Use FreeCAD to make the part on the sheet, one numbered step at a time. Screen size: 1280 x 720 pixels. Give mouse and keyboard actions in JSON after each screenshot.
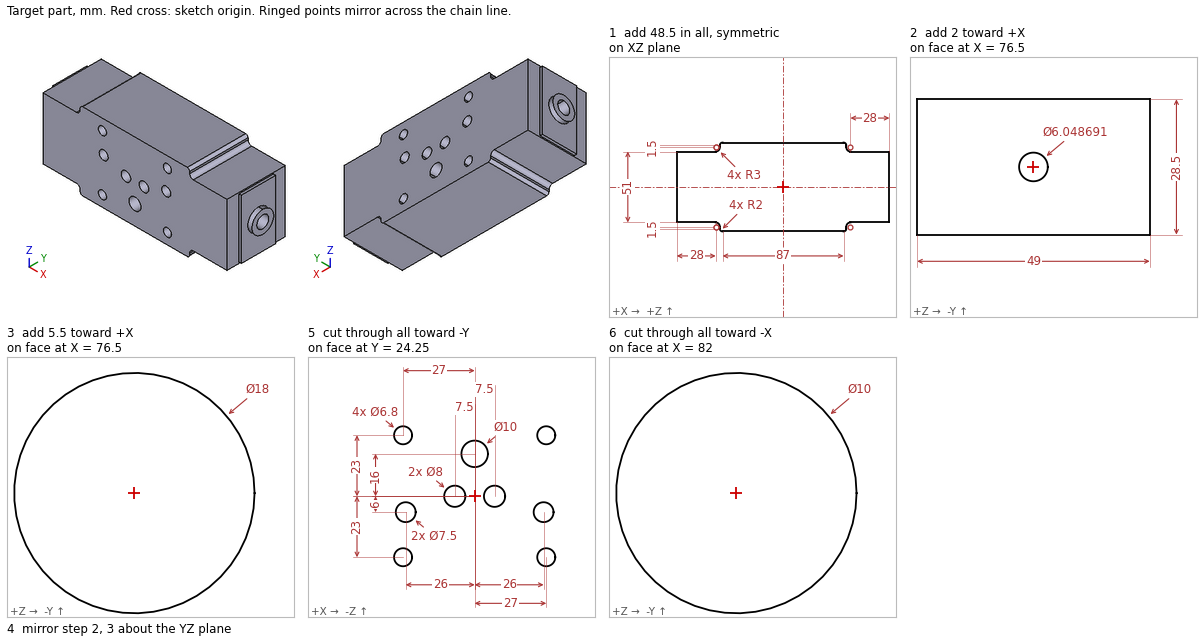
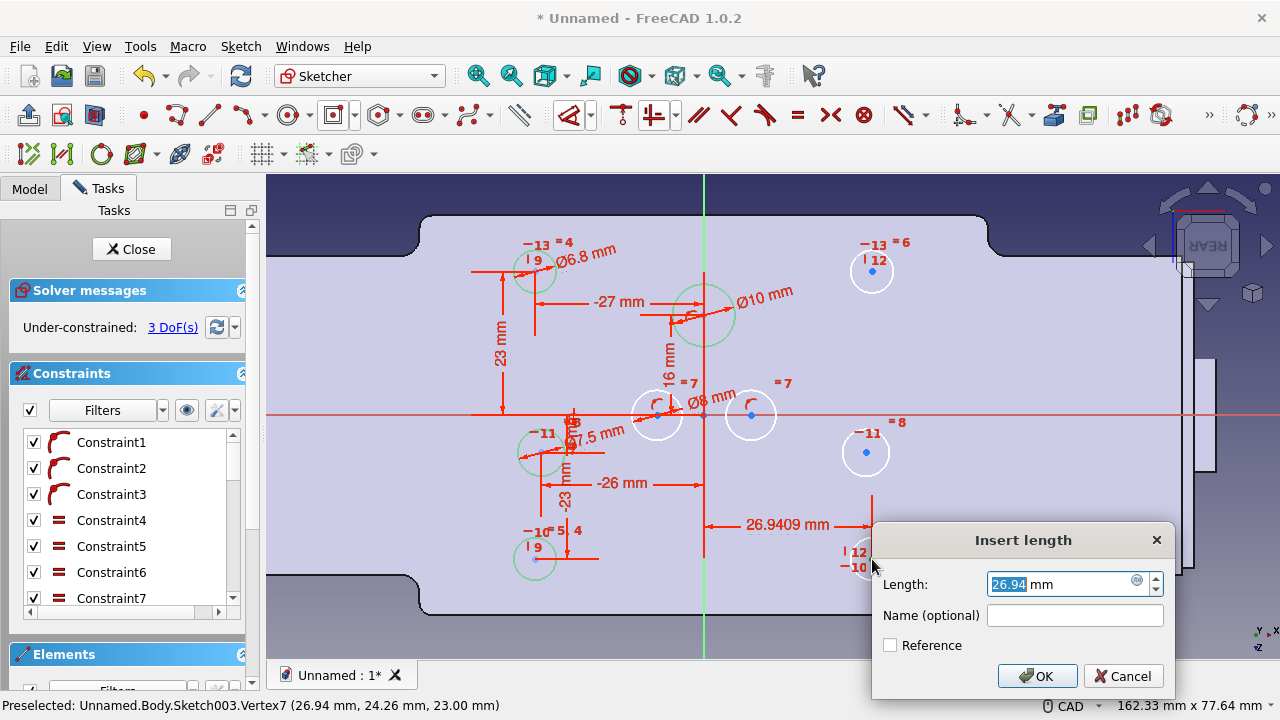
{"action": "type", "text": "27"}
{"action": "key", "text": "Return"}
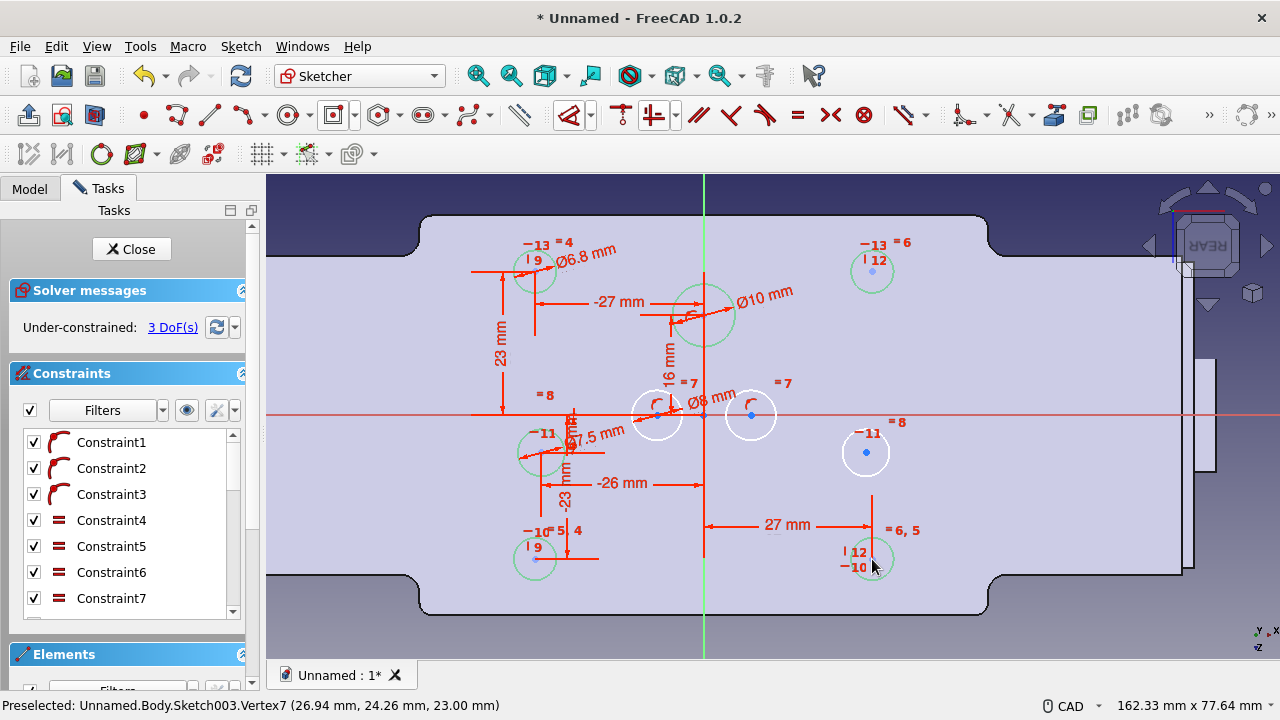
{"action": "left_click", "coordinate": [866, 453]}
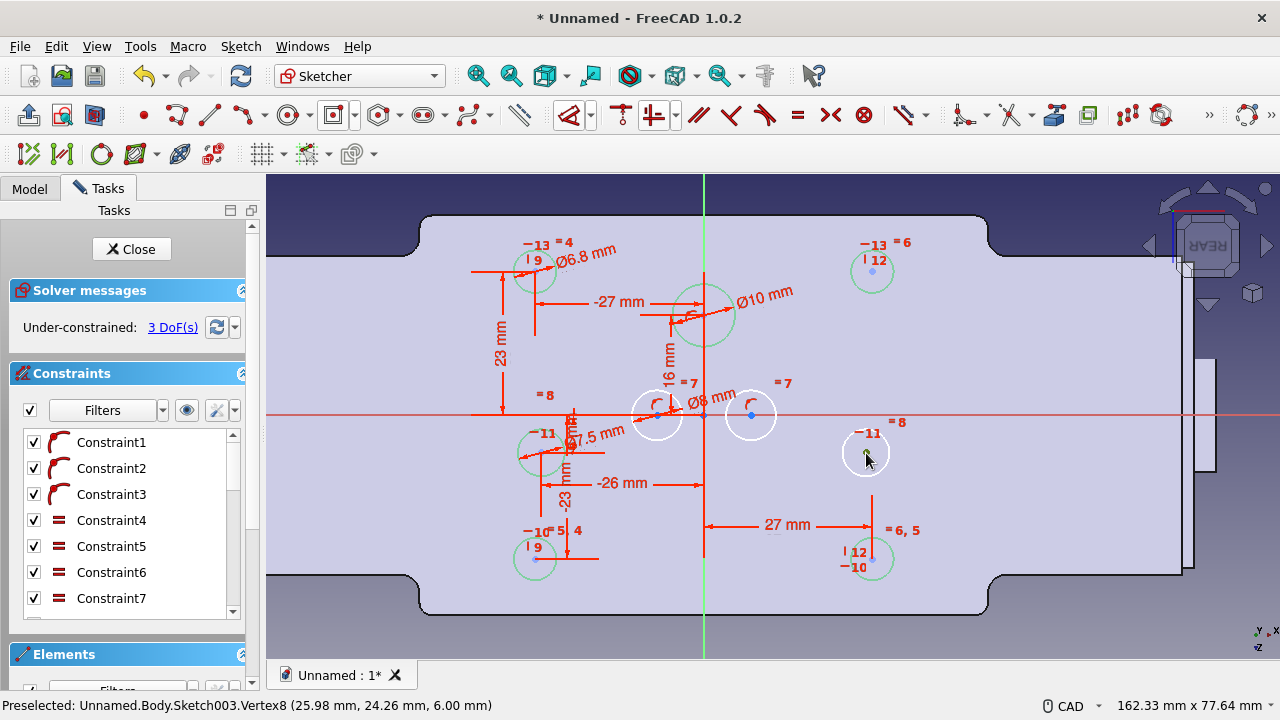
{"action": "key", "text": "l"}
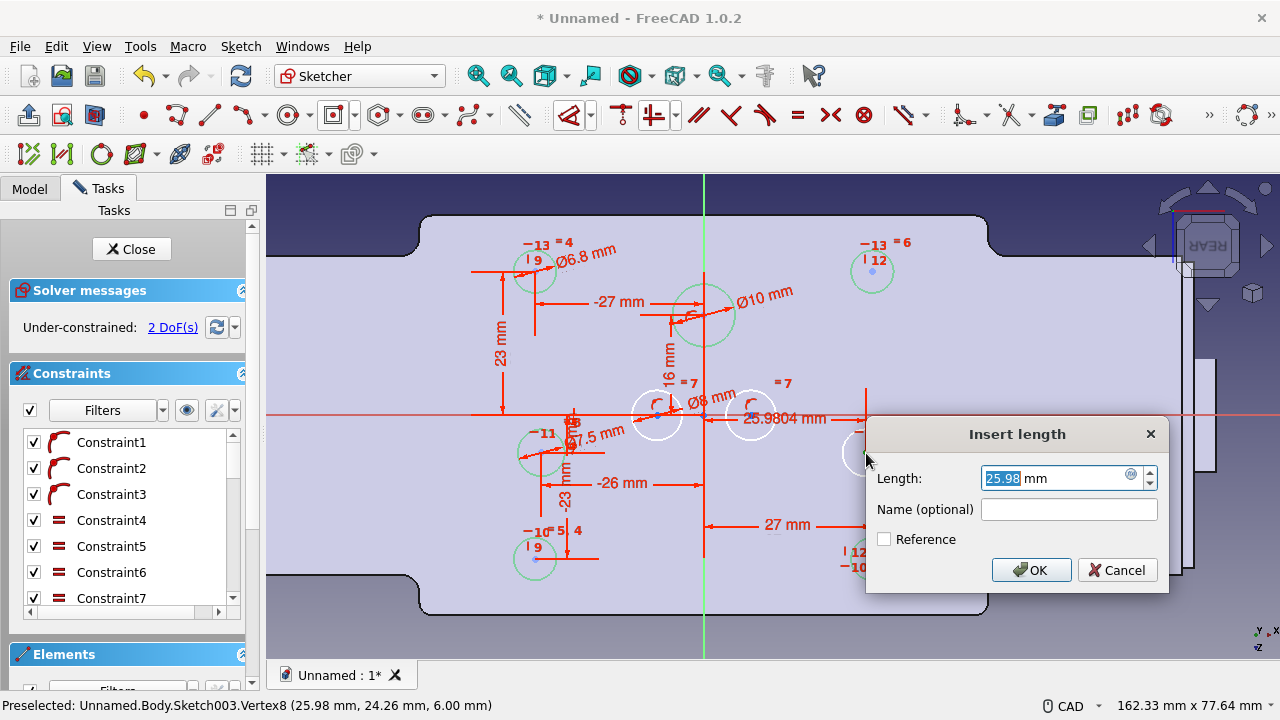
{"action": "type", "text": "26"}
{"action": "key", "text": "Return"}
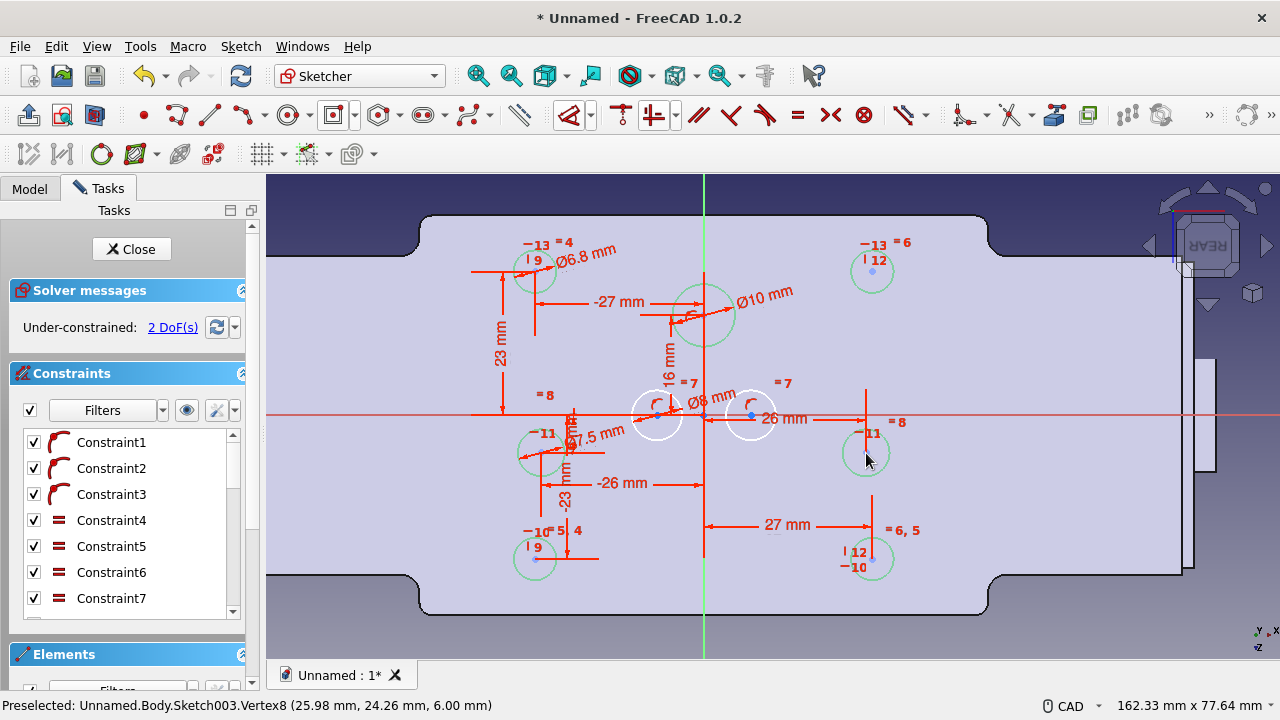
{"action": "left_click", "coordinate": [657, 415]}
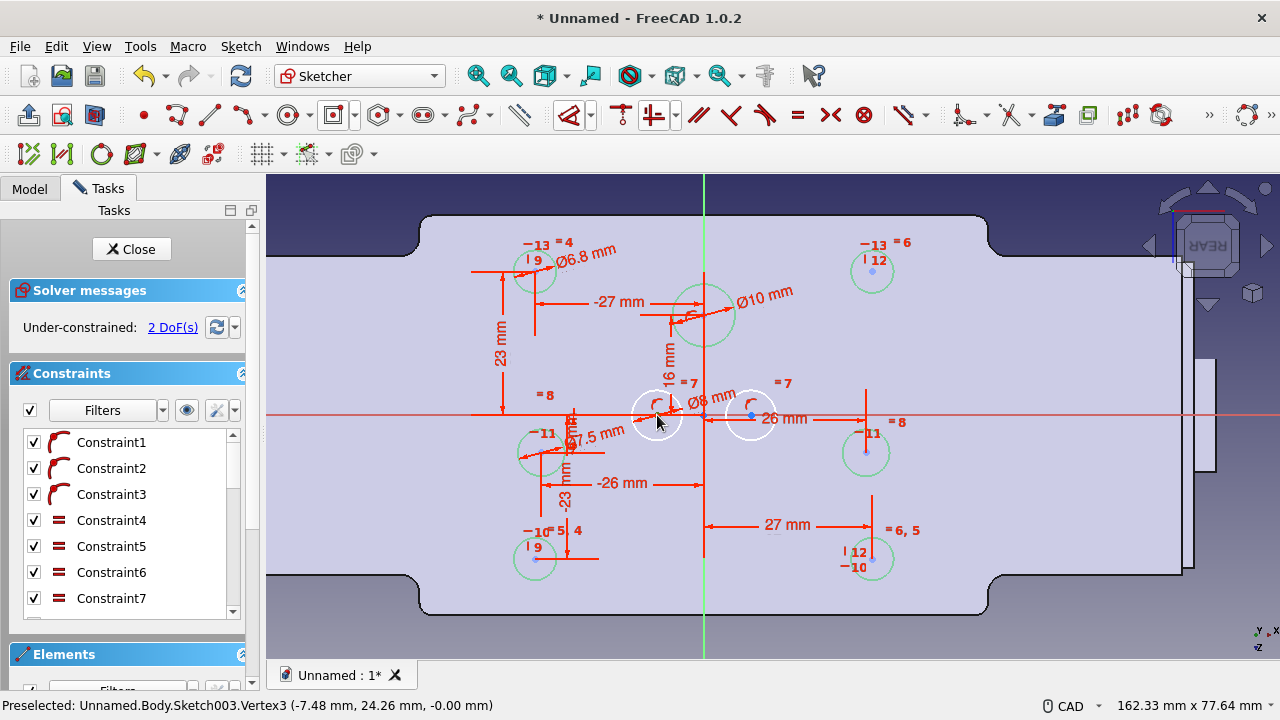
{"action": "key", "text": "l"}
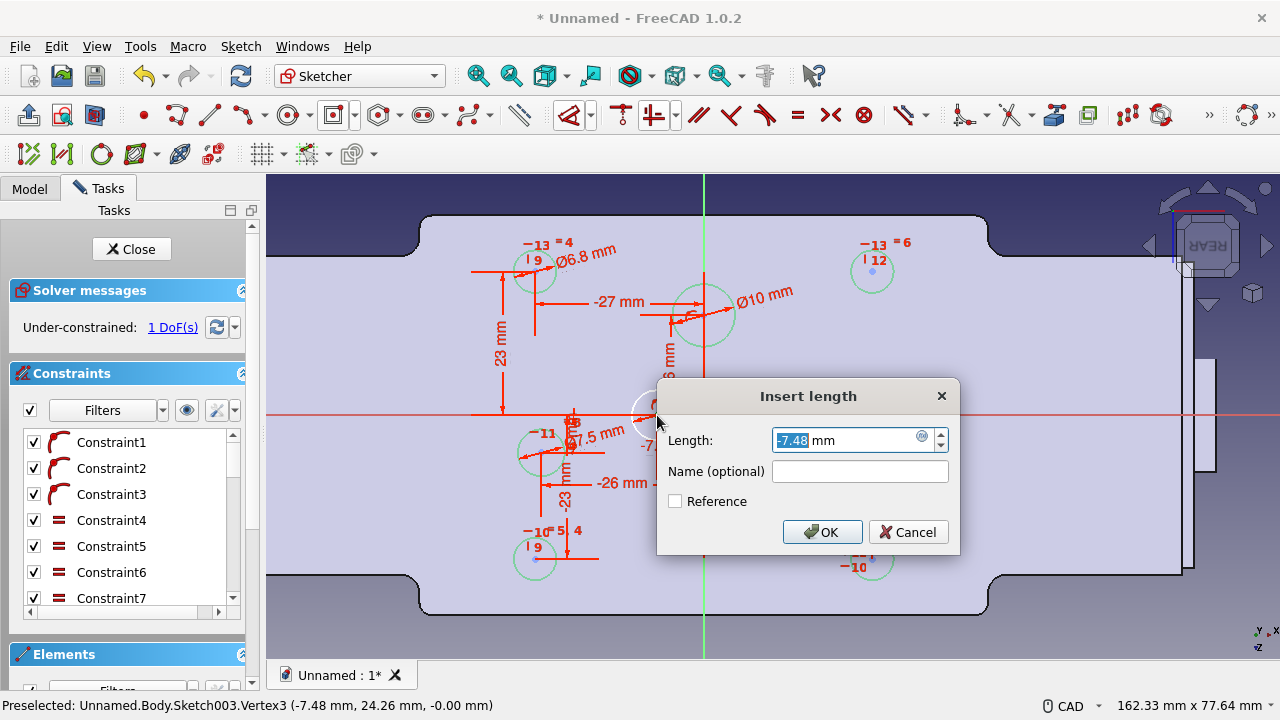
{"action": "type", "text": "-7.5"}
{"action": "key", "text": "Return"}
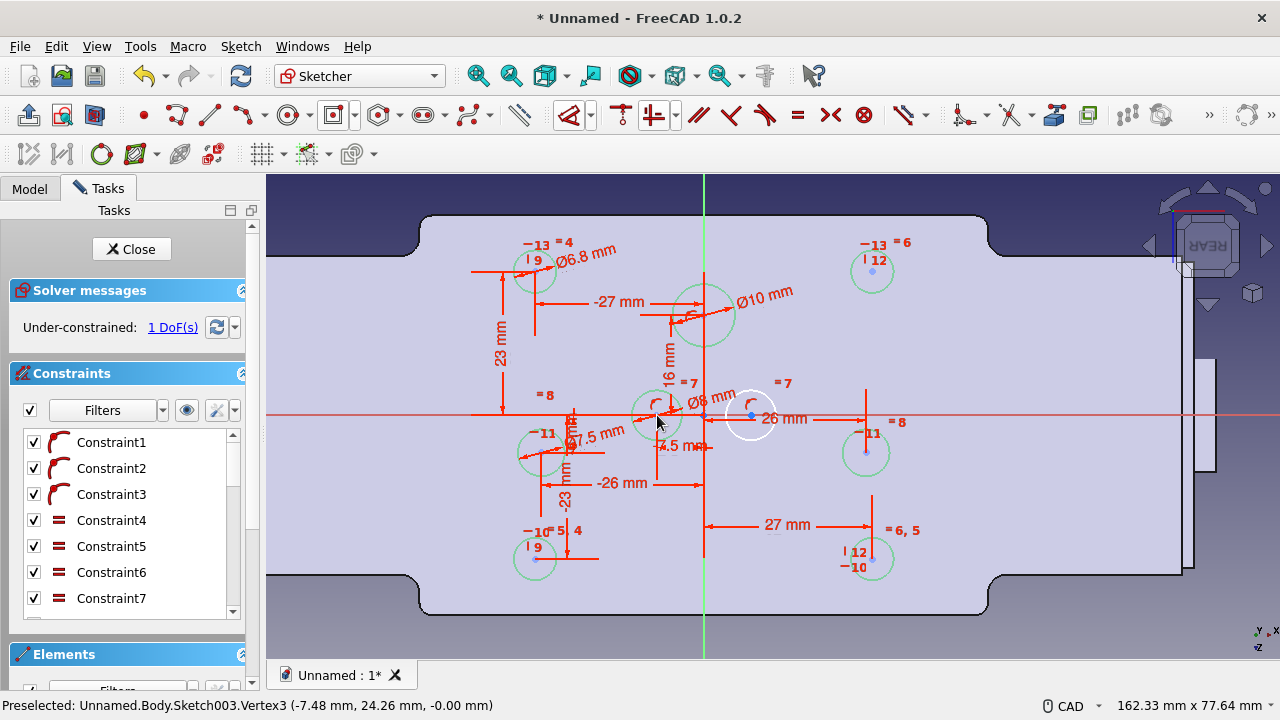
{"action": "left_click", "coordinate": [751, 415]}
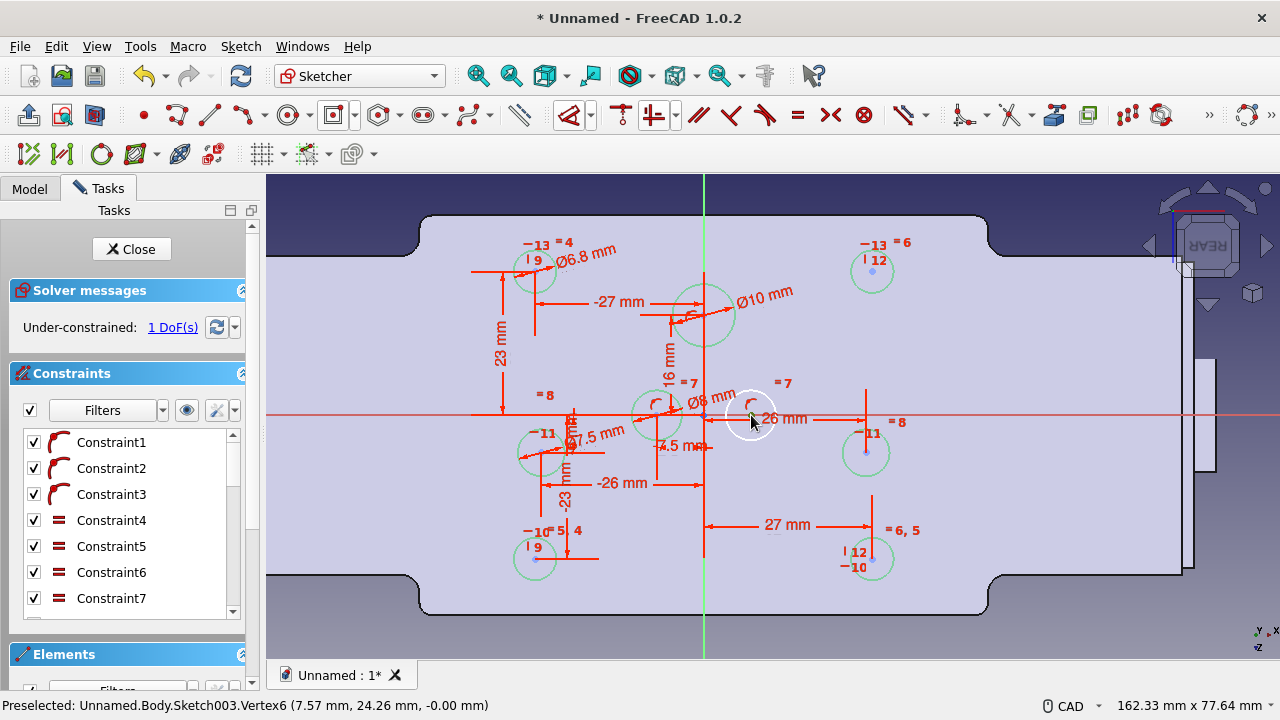
{"action": "key", "text": "l"}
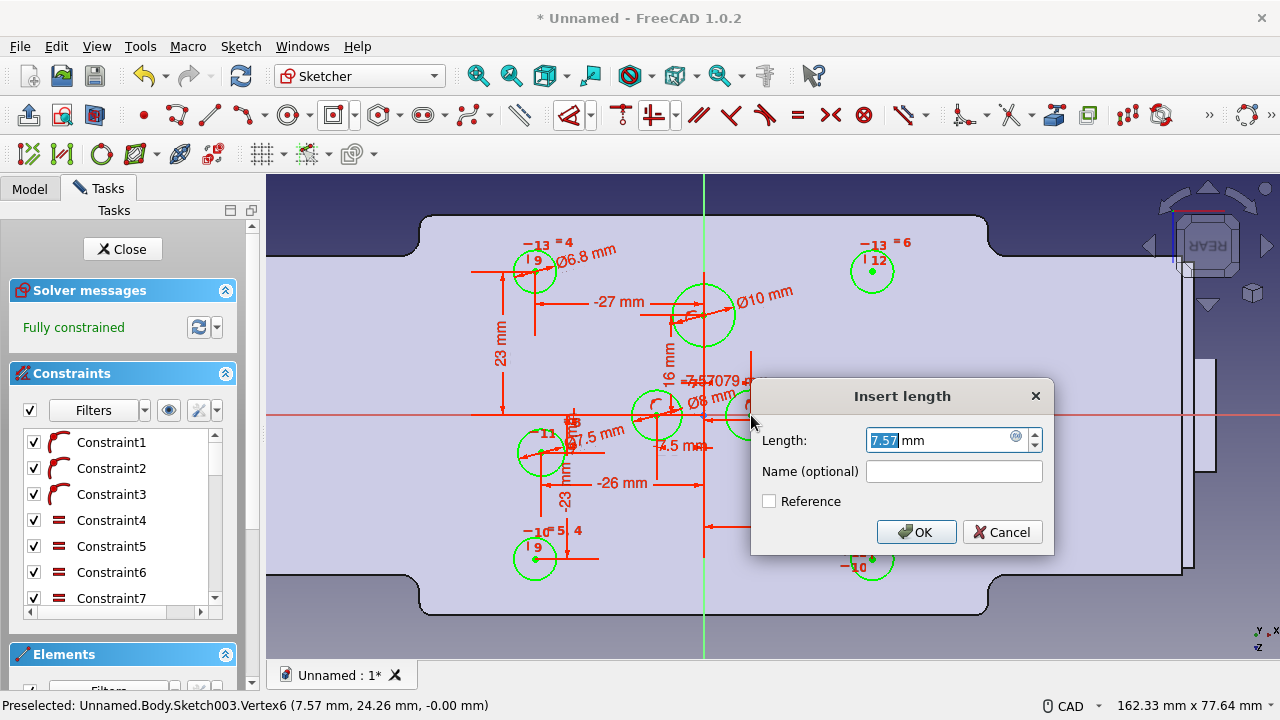
{"action": "type", "text": "7.5"}
{"action": "key", "text": "Return"}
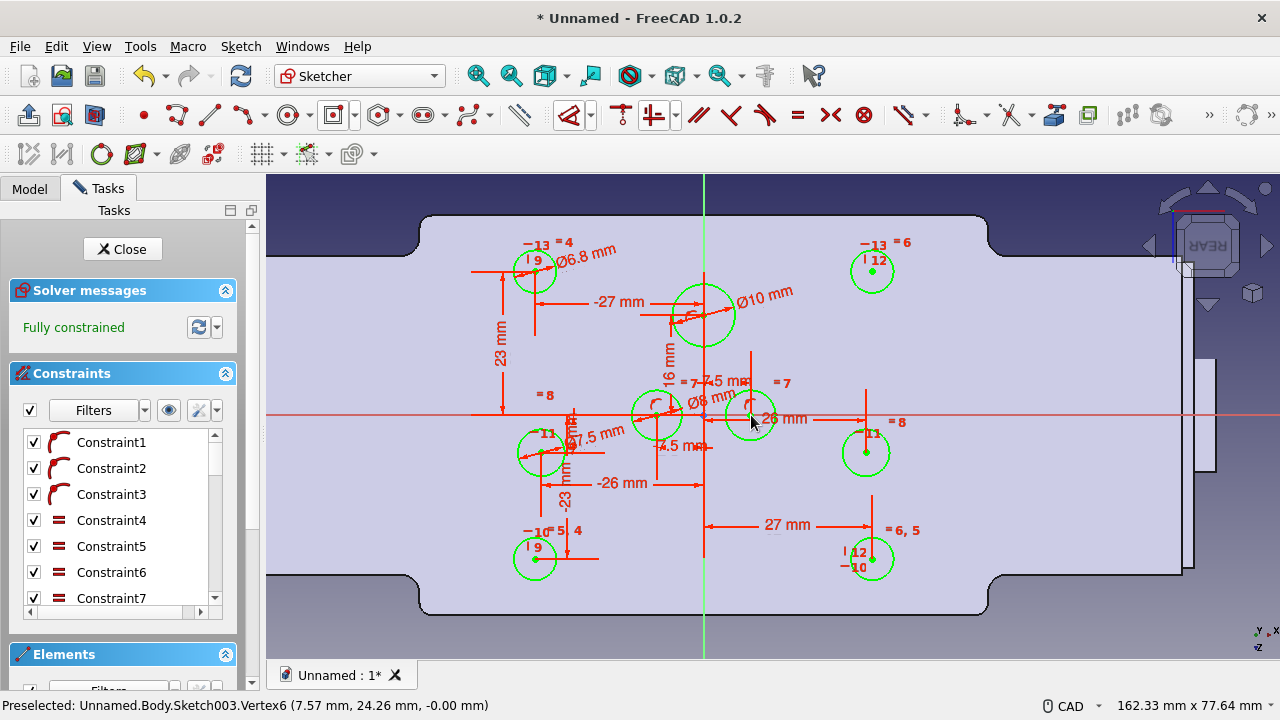
{"action": "left_click", "coordinate": [123, 249]}